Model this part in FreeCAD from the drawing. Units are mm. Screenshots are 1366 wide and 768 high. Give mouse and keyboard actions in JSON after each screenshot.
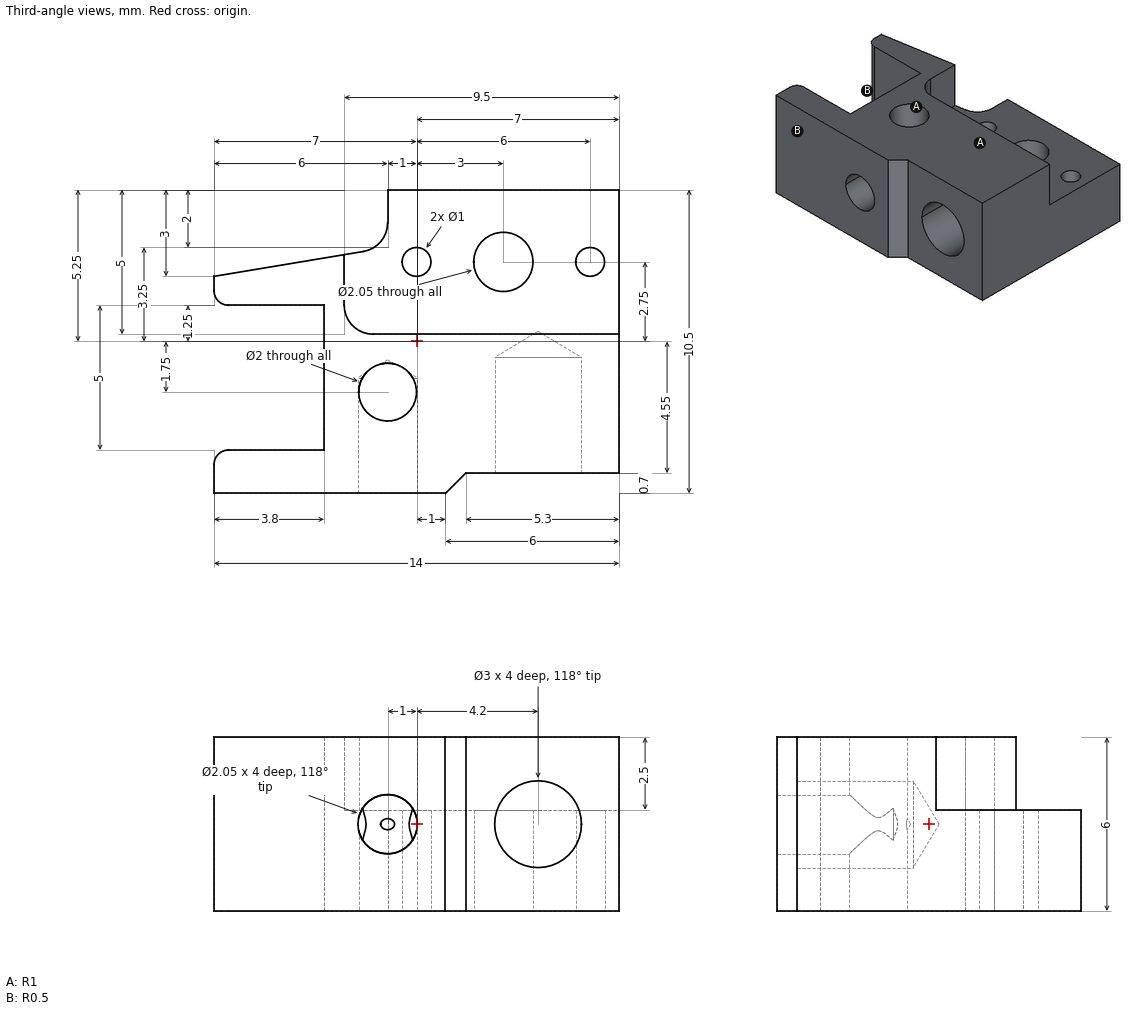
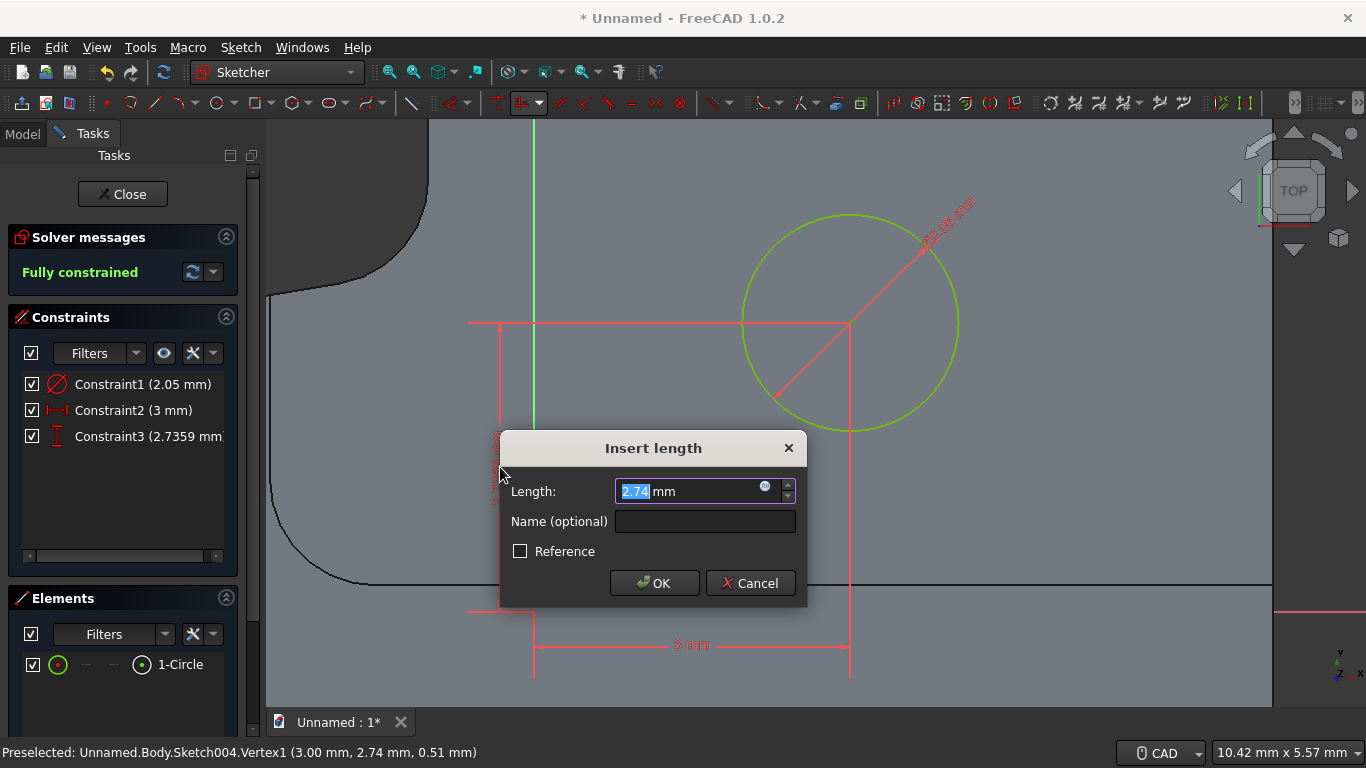
{"action": "type", "text": "2.75"}
{"action": "key", "text": "Return"}
{"action": "key", "text": "Escape"}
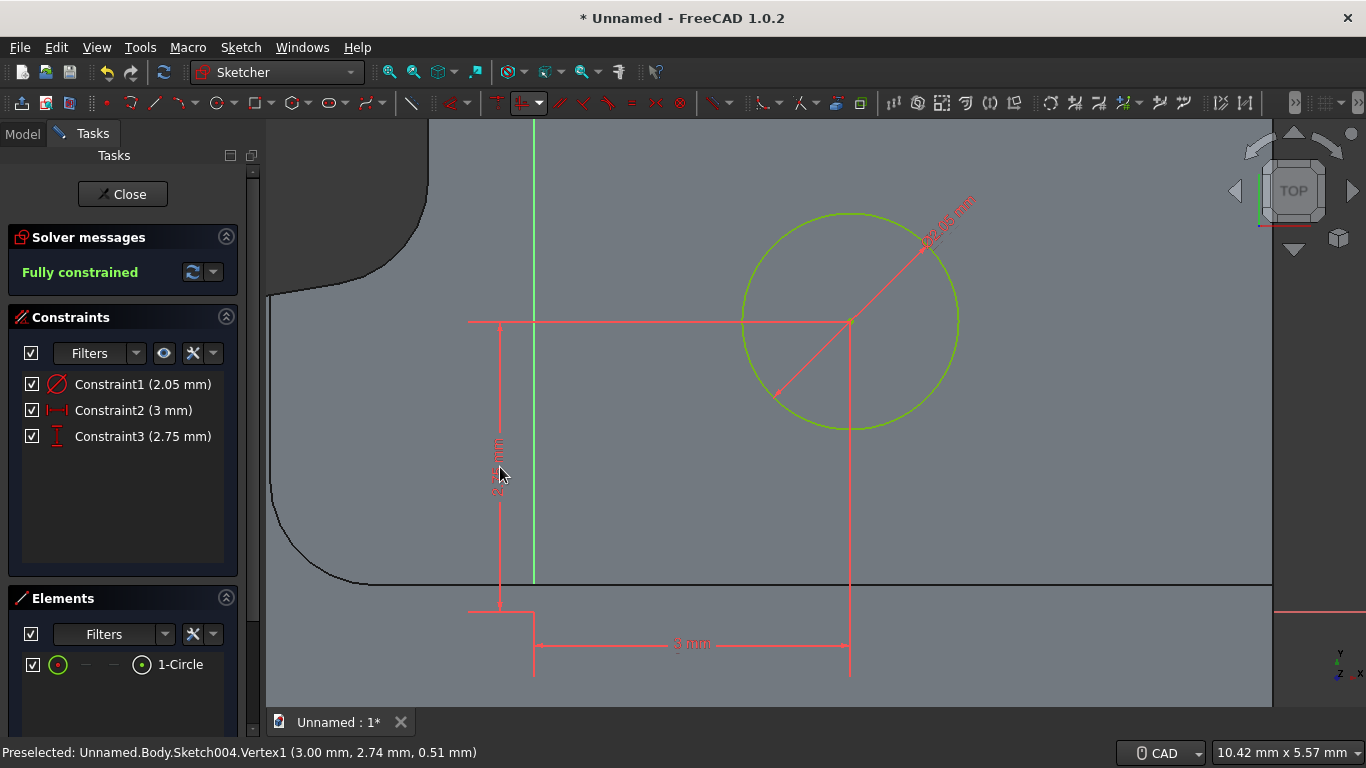
{"action": "left_click", "coordinate": [123, 194]}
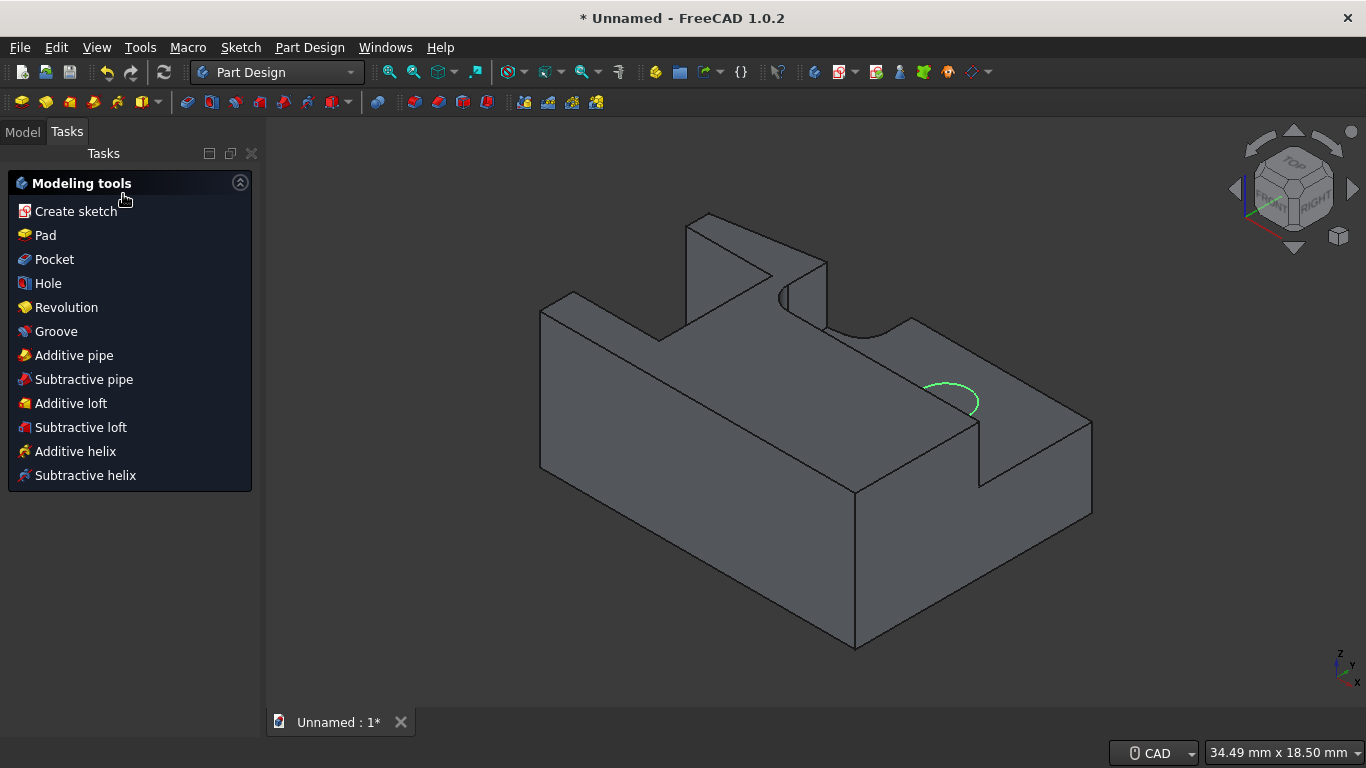
{"action": "left_click", "coordinate": [212, 102]}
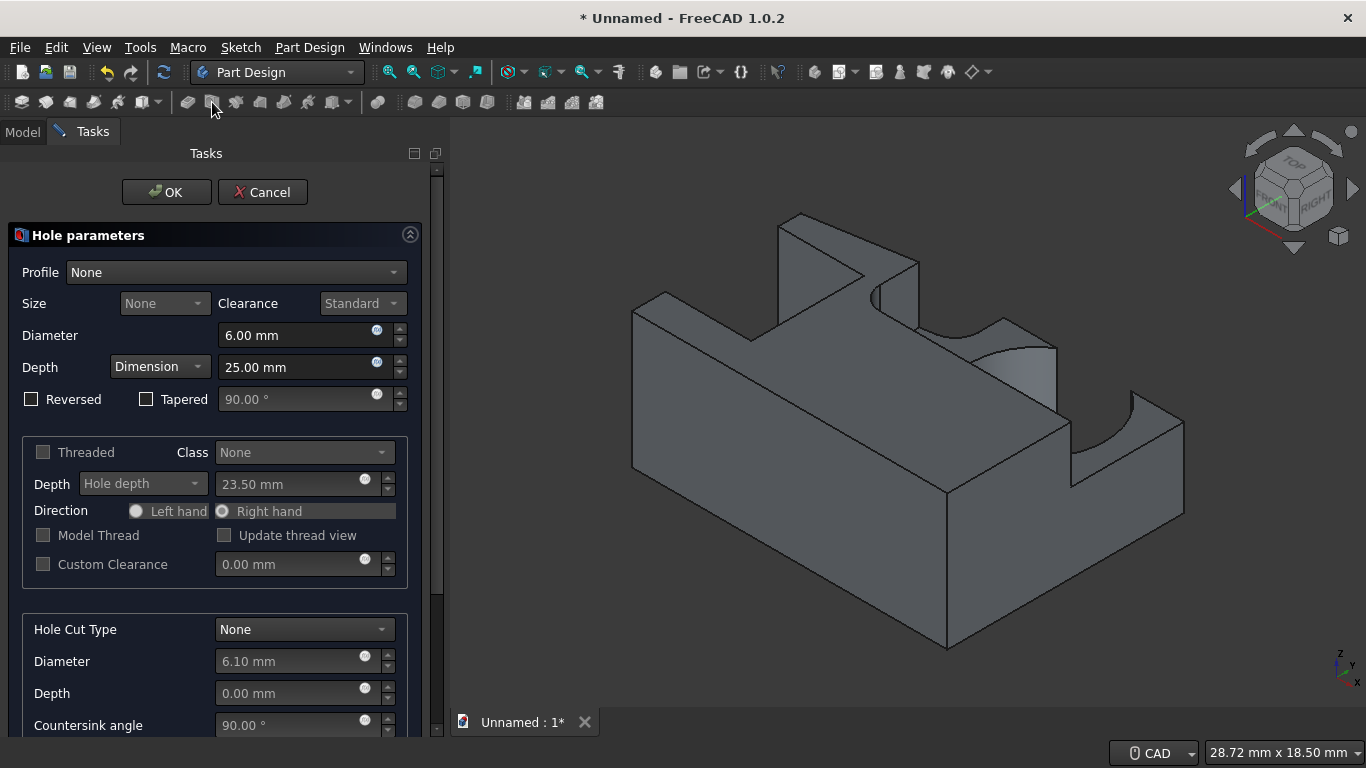
{"action": "triple_click", "coordinate": [305, 335]}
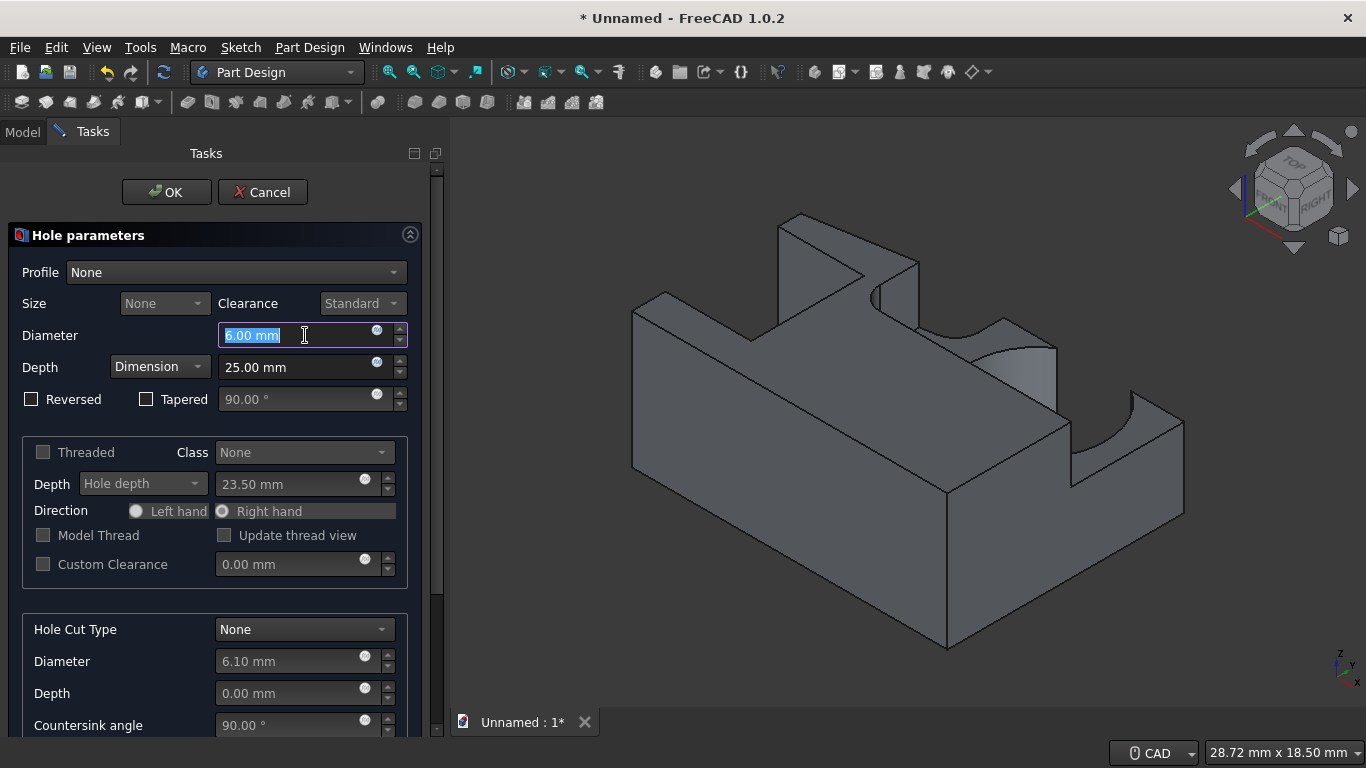
{"action": "type", "text": "2.05"}
{"action": "key", "text": "Tab"}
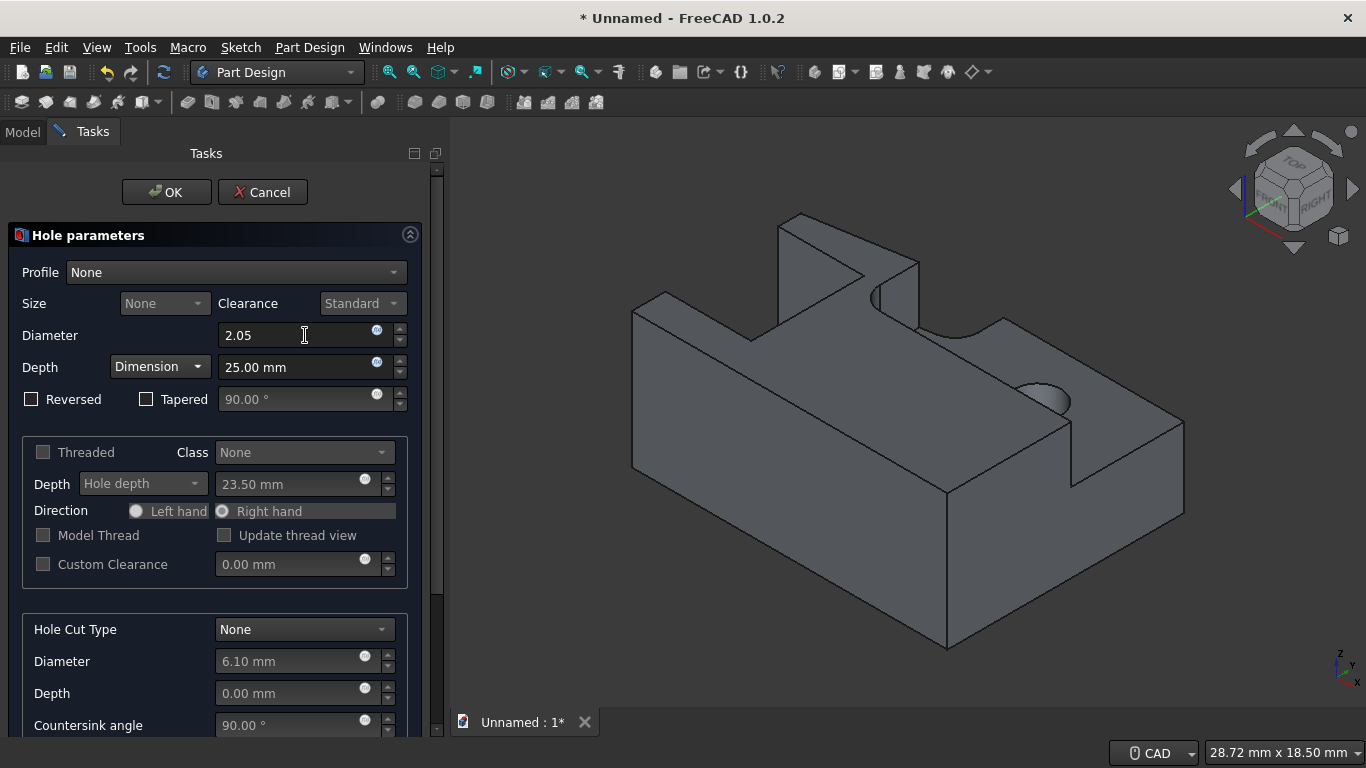
{"action": "left_click", "coordinate": [161, 366]}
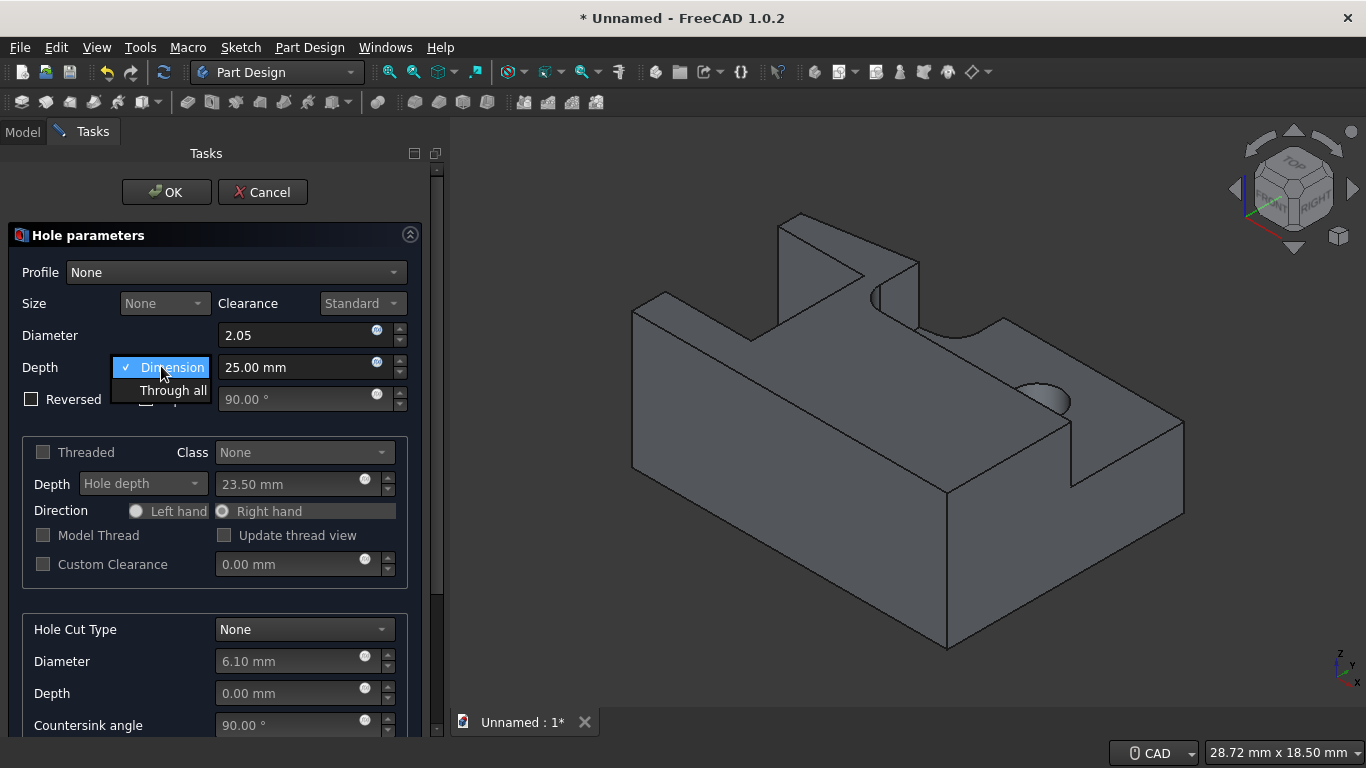
{"action": "left_click", "coordinate": [160, 390]}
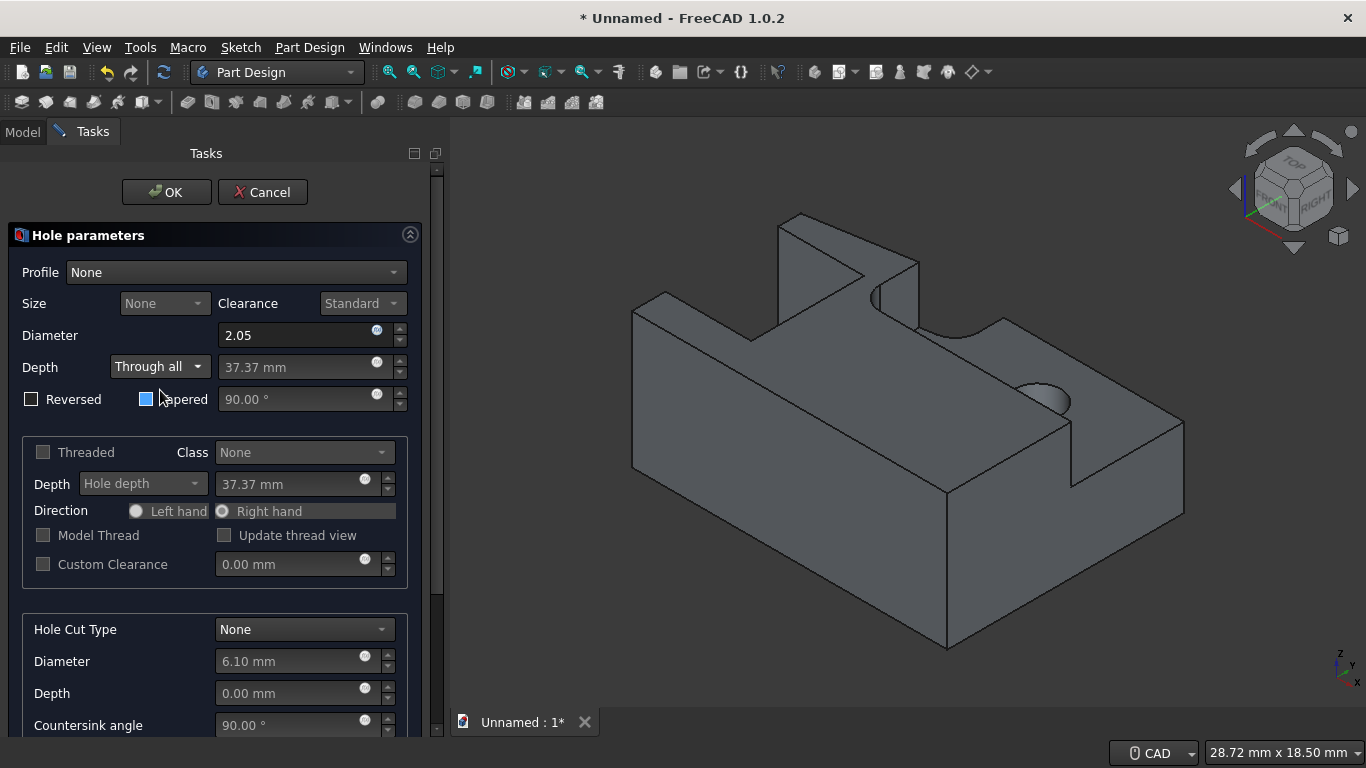
{"action": "left_click", "coordinate": [167, 192]}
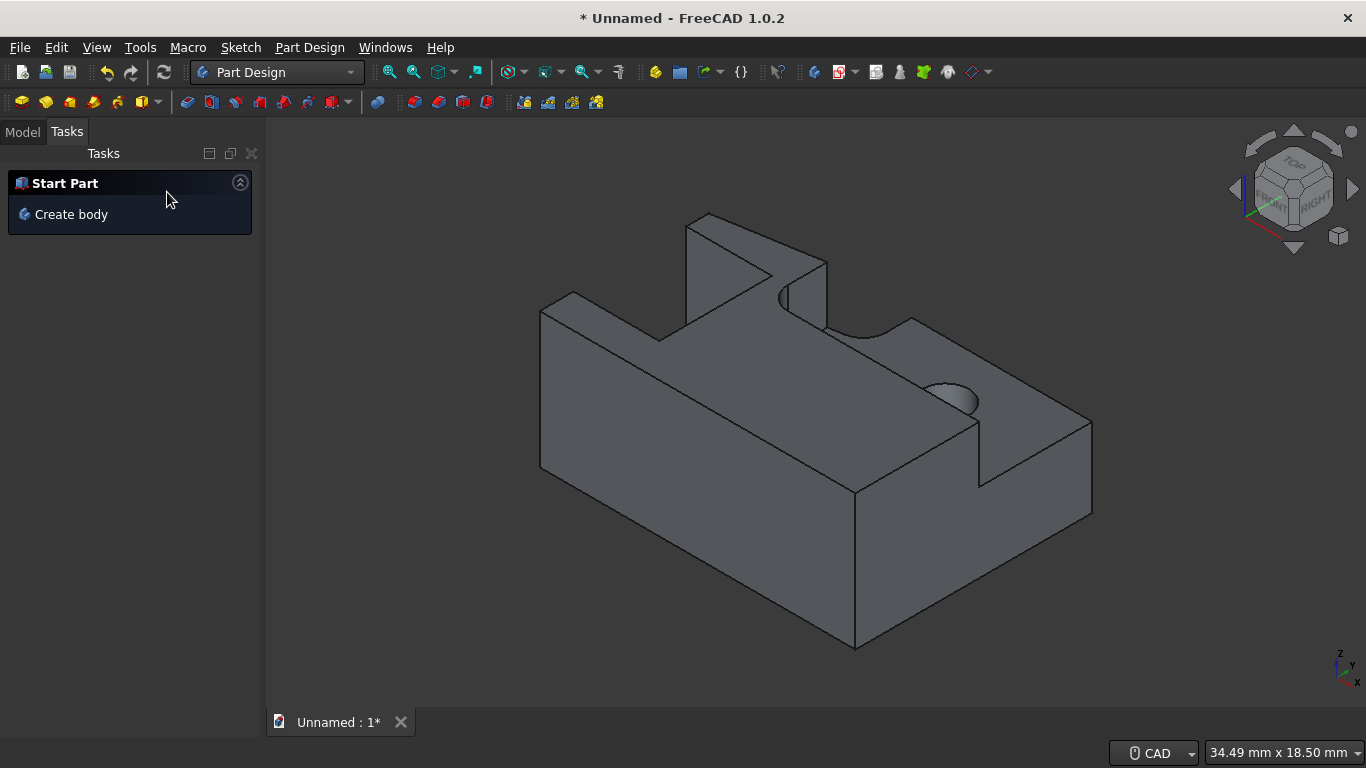
{"action": "left_click", "coordinate": [914, 365]}